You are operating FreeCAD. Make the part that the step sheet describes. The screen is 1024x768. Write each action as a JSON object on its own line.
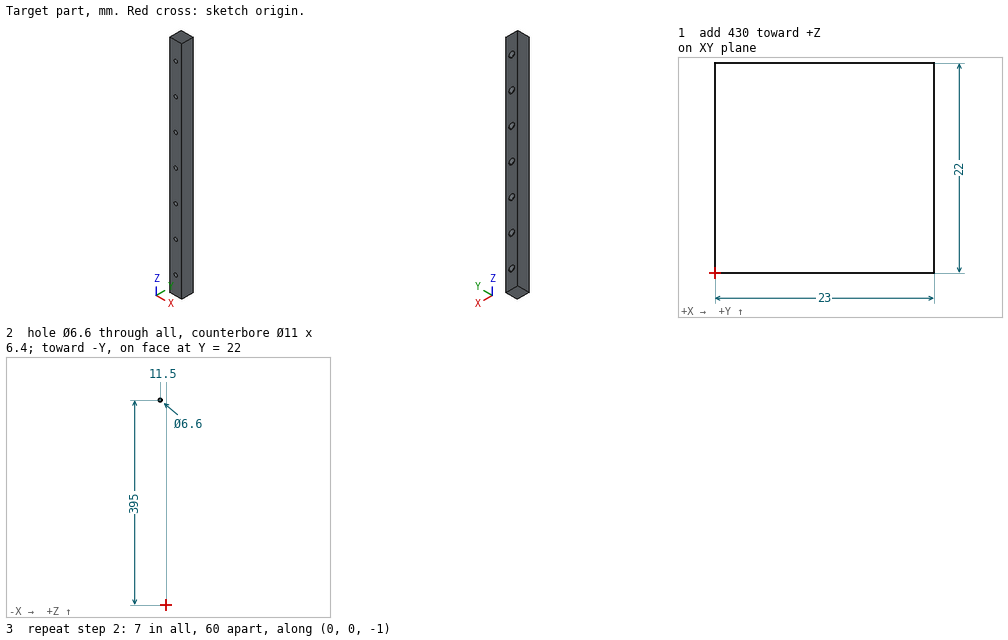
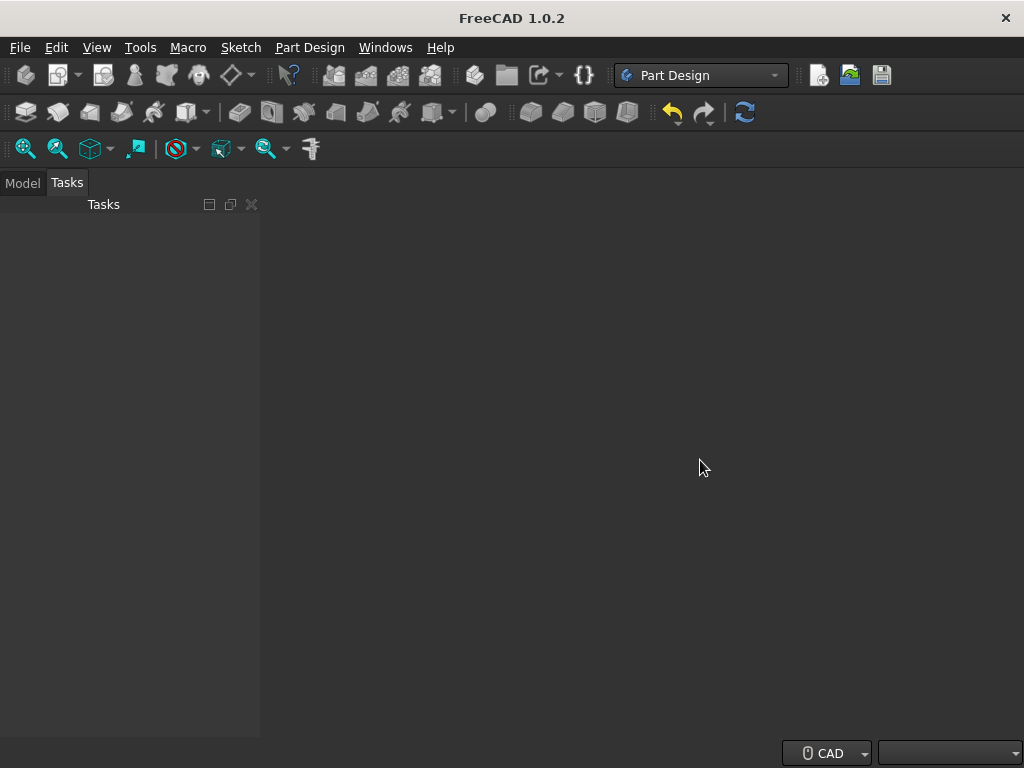
{"action": "left_click", "coordinate": [818, 76]}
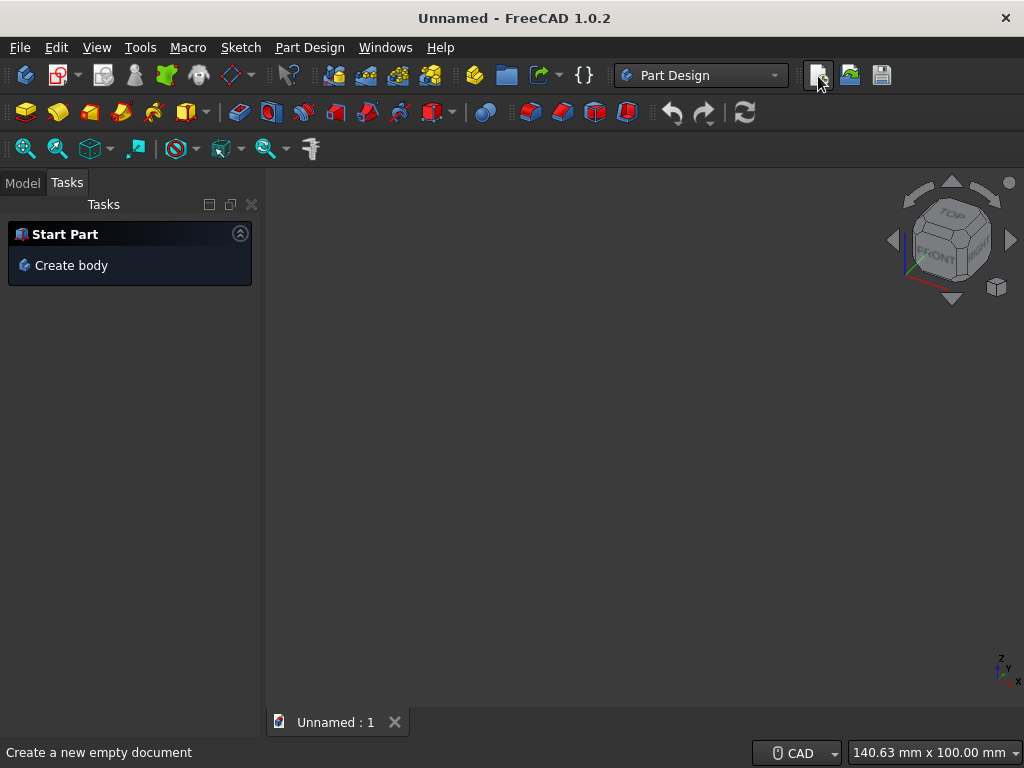
{"action": "left_click", "coordinate": [58, 76]}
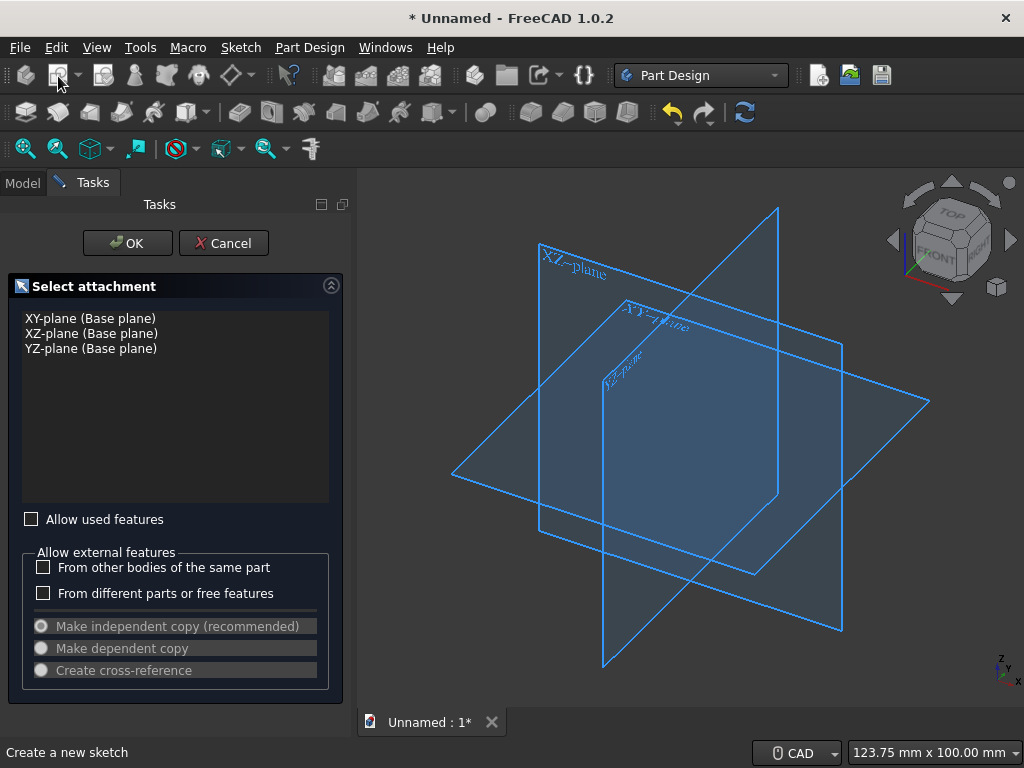
{"action": "left_click", "coordinate": [82, 318]}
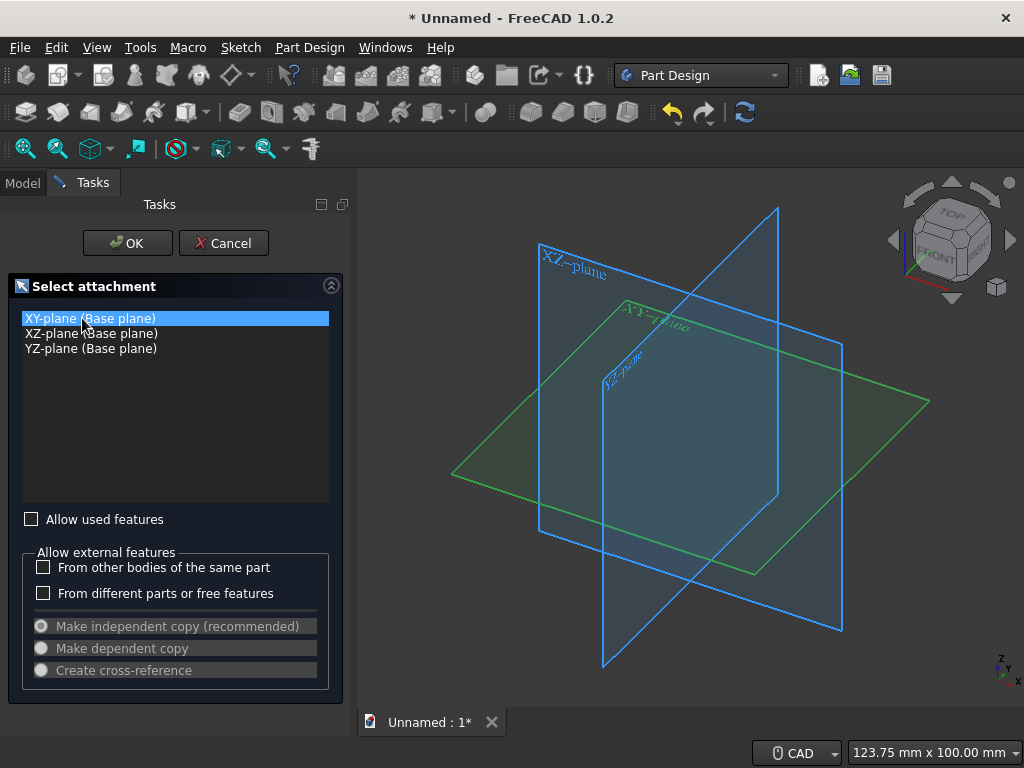
{"action": "left_click", "coordinate": [128, 243]}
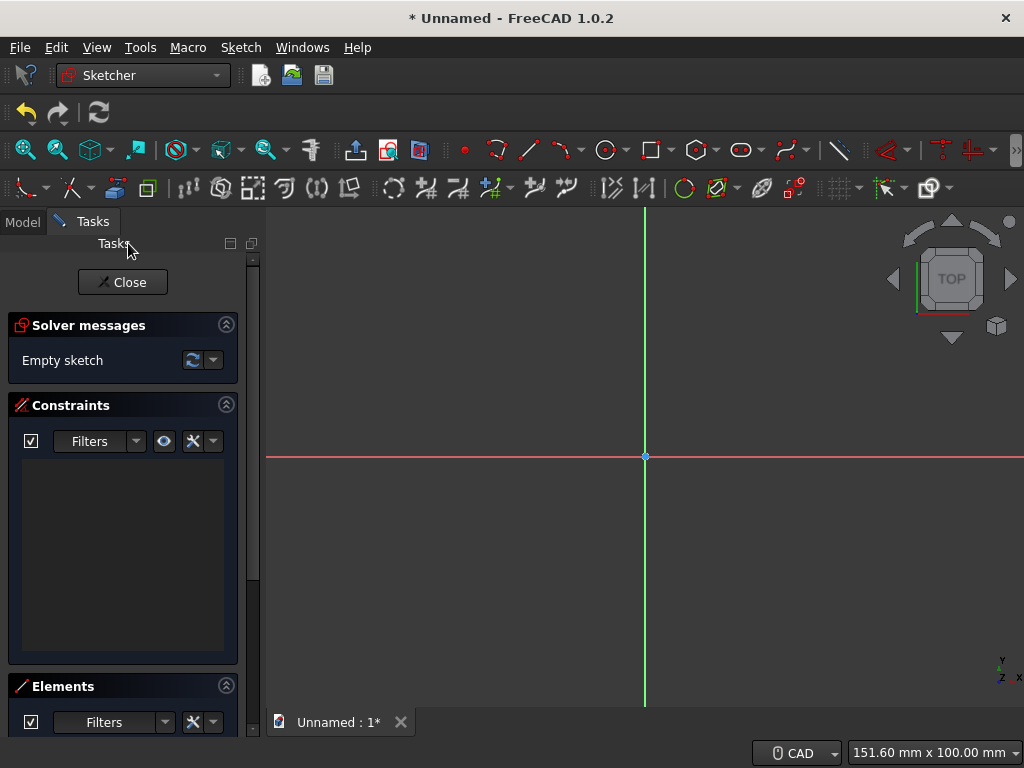
{"action": "scroll", "coordinate": [776, 370], "scroll_direction": "up", "scroll_amount": 5}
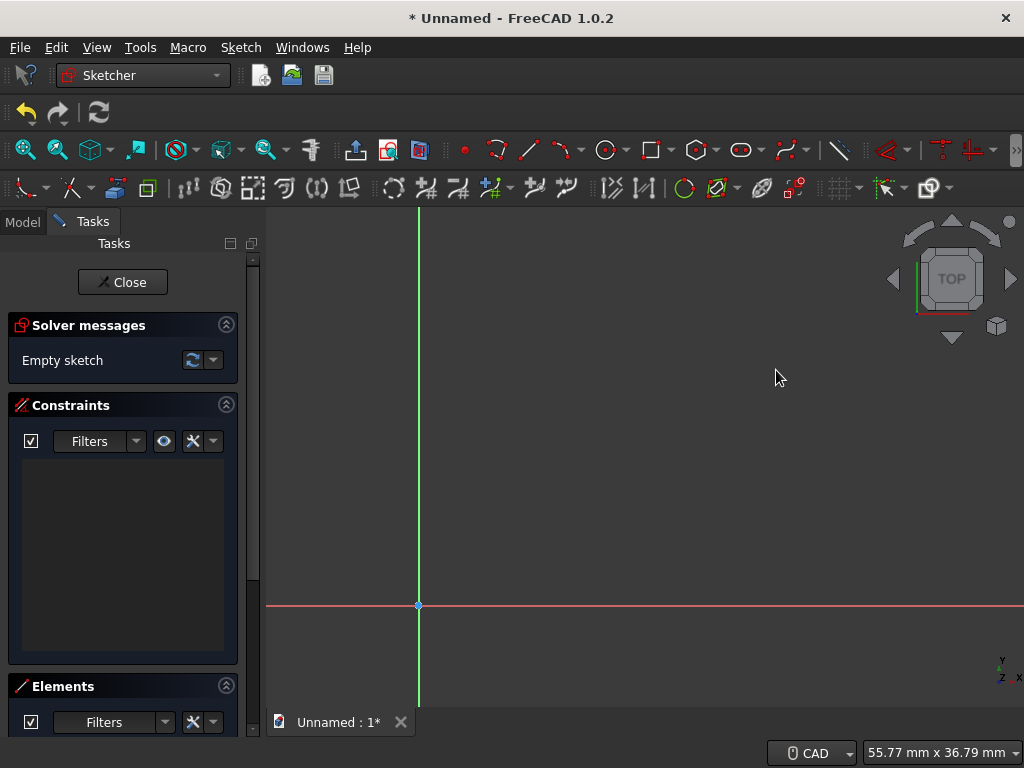
{"action": "left_click", "coordinate": [652, 150]}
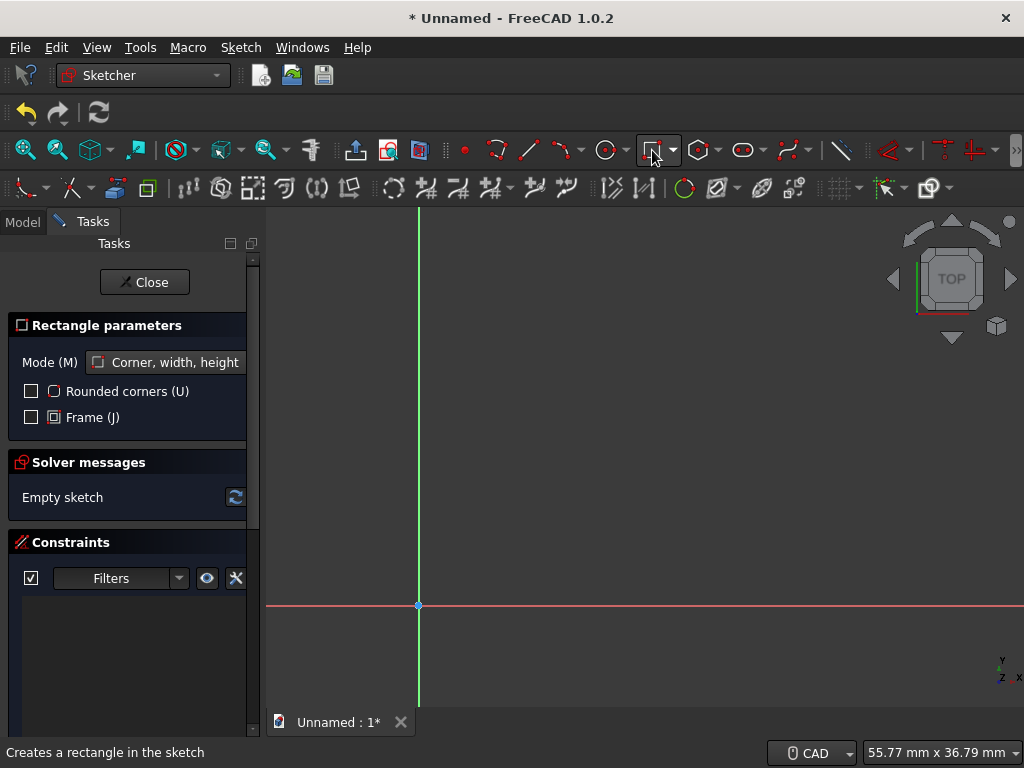
{"action": "left_click", "coordinate": [419, 606]}
{"action": "mouse_move", "coordinate": [731, 307]}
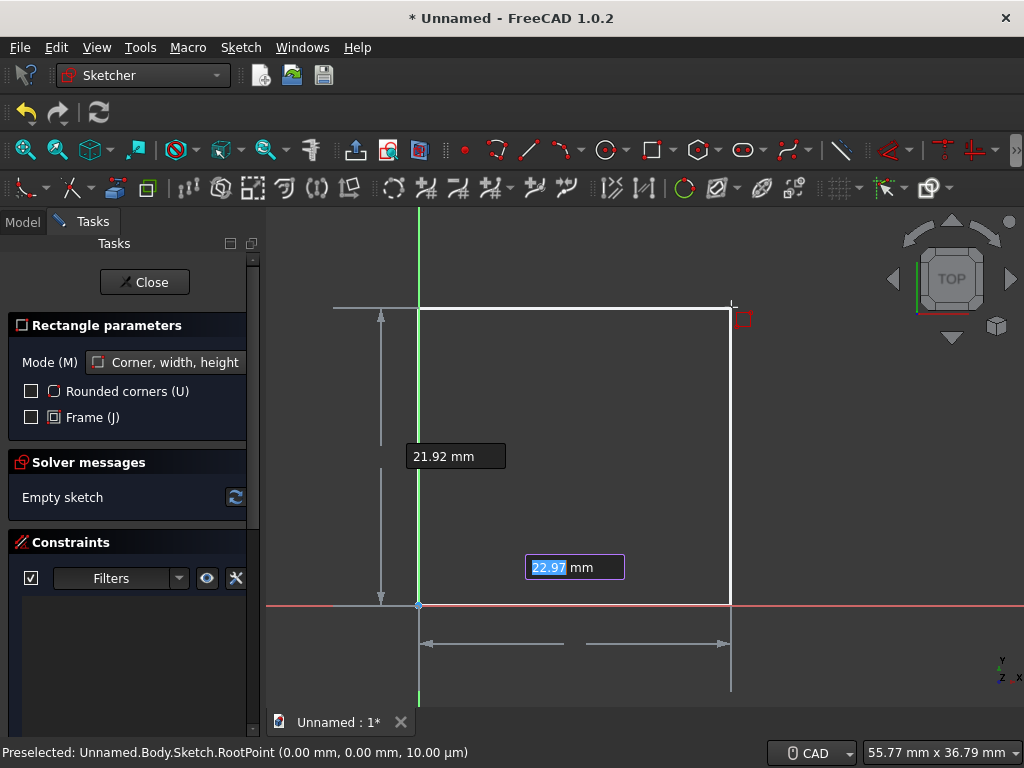
{"action": "type", "text": "23"}
{"action": "key", "text": "Tab"}
{"action": "type", "text": "22"}
{"action": "key", "text": "Return"}
{"action": "key", "text": "Escape"}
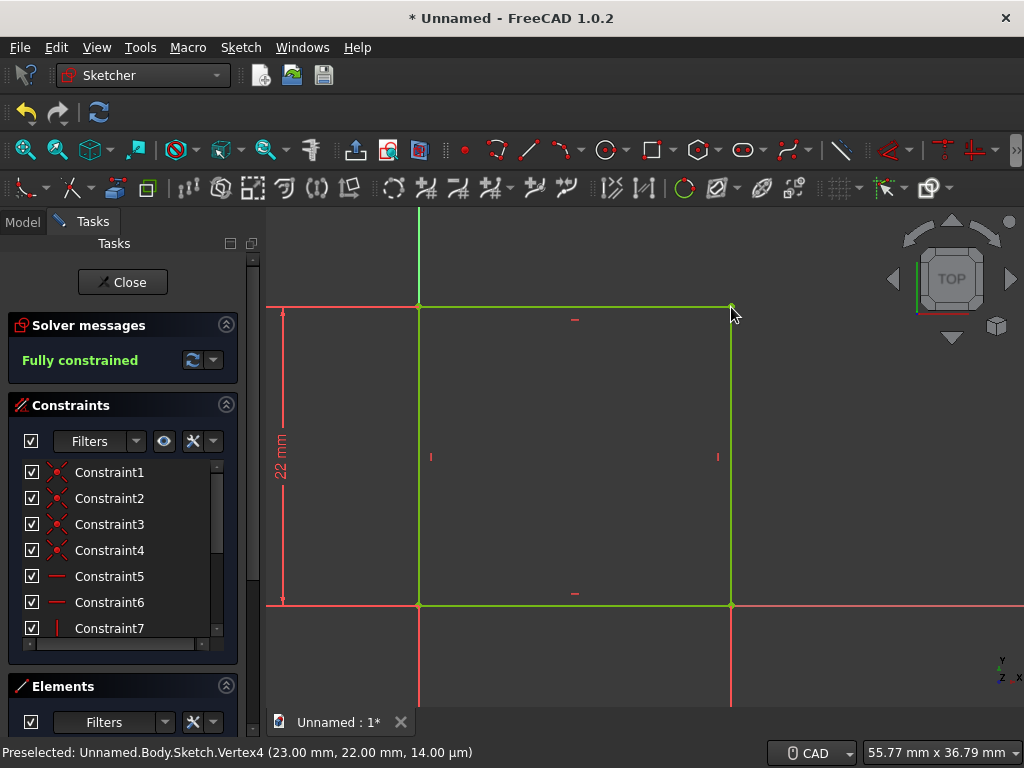
{"action": "left_click", "coordinate": [123, 282]}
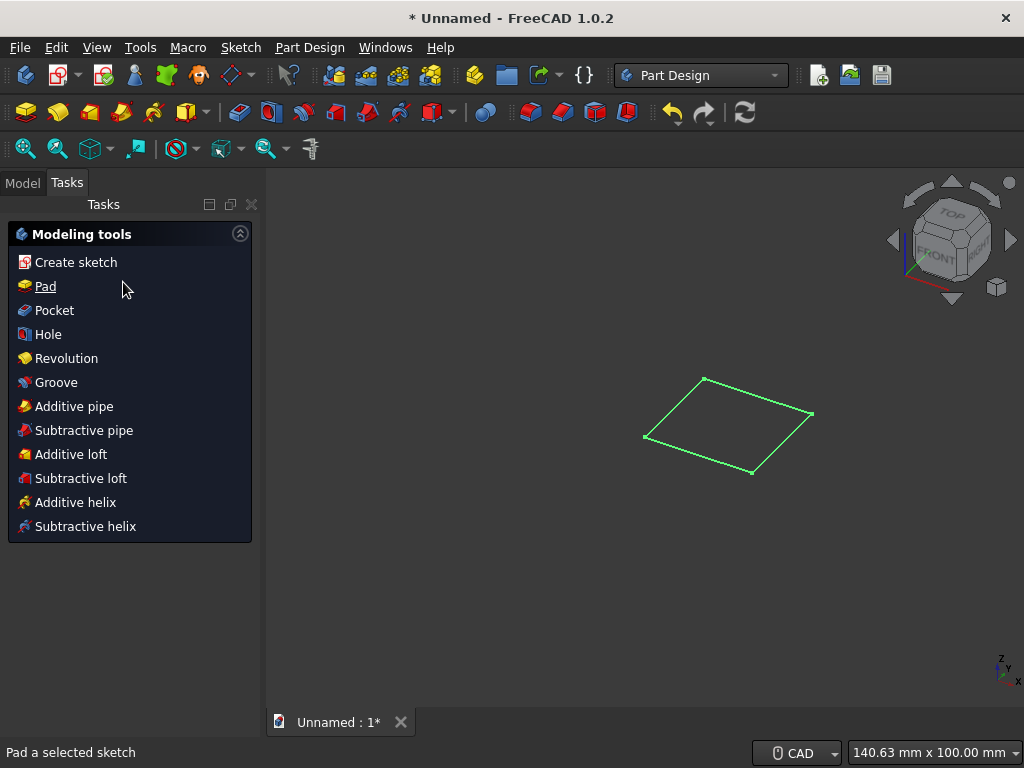
{"action": "left_click", "coordinate": [26, 112]}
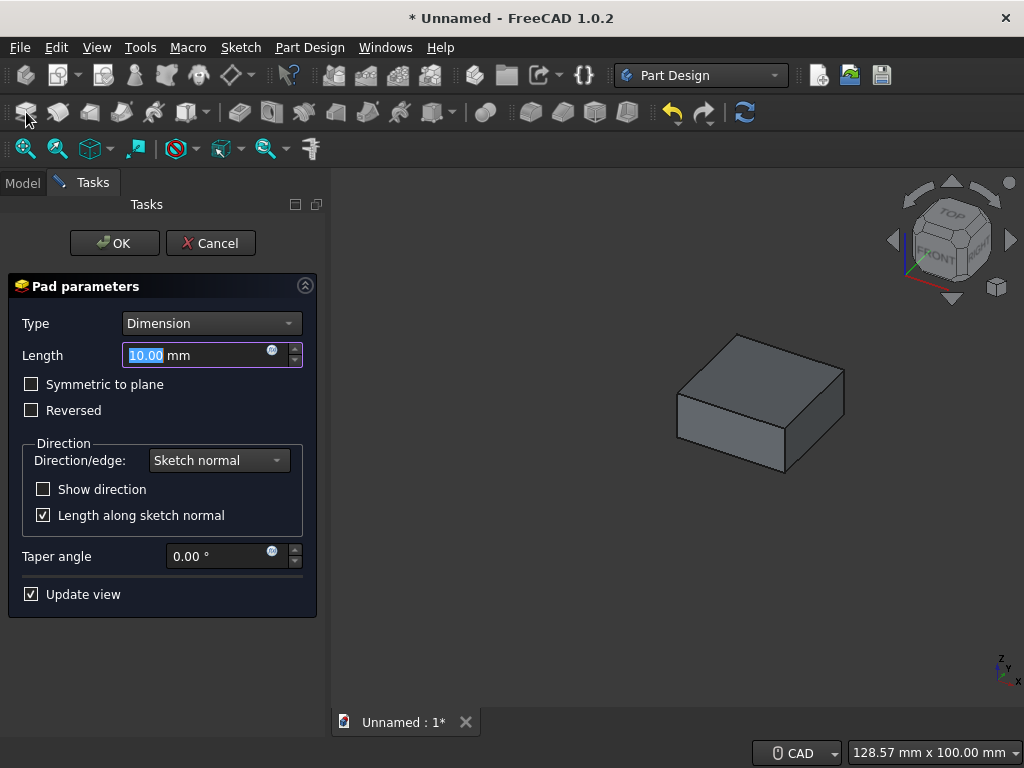
{"action": "type", "text": "430"}
{"action": "key", "text": "Tab"}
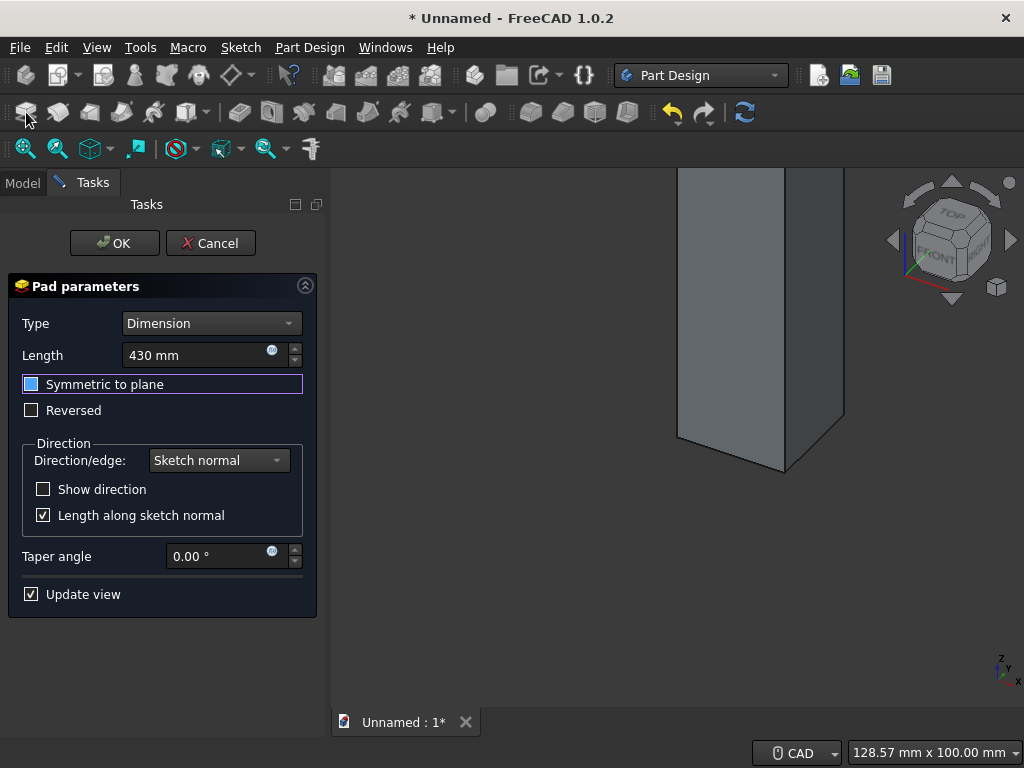
{"action": "left_click", "coordinate": [115, 243]}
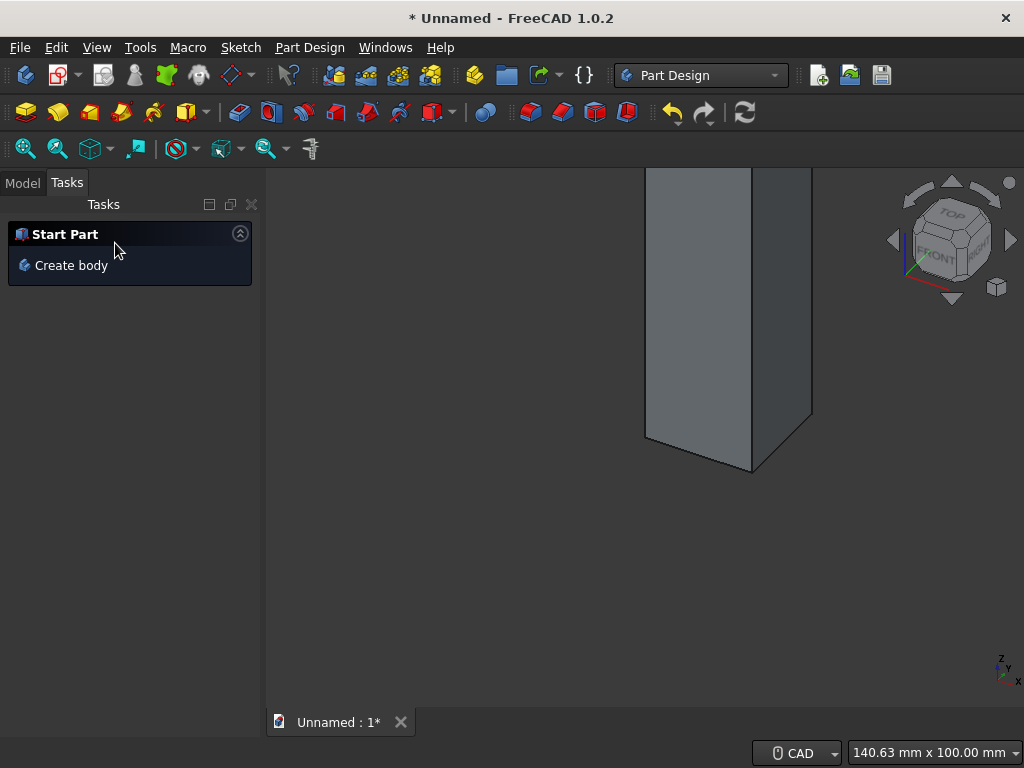
{"action": "left_click", "coordinate": [26, 150]}